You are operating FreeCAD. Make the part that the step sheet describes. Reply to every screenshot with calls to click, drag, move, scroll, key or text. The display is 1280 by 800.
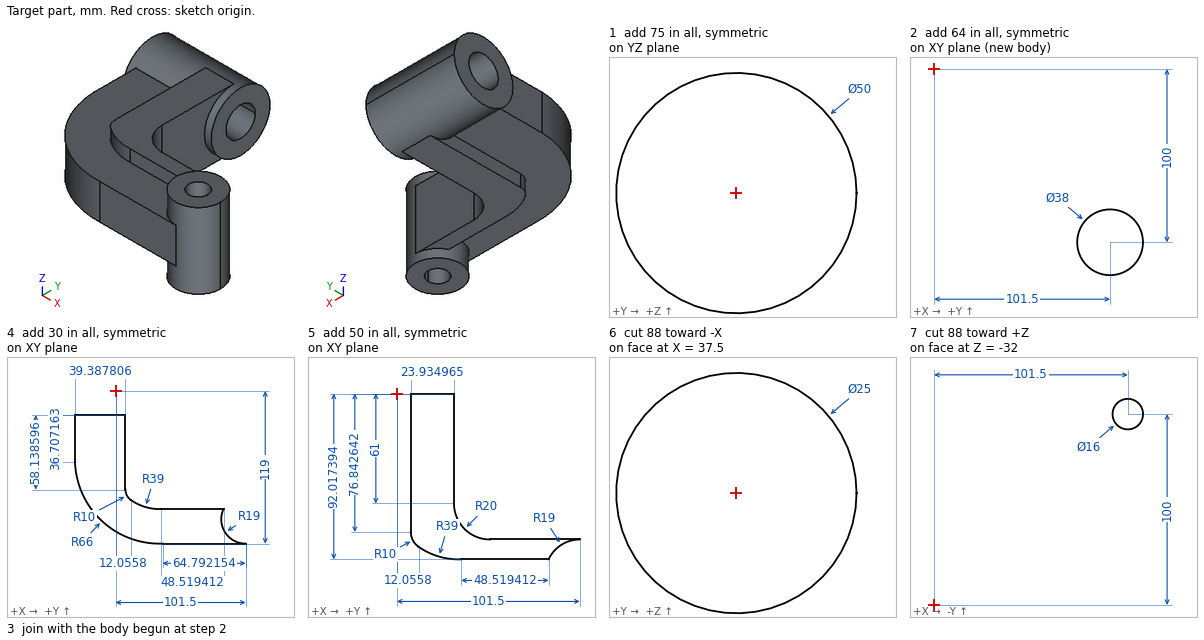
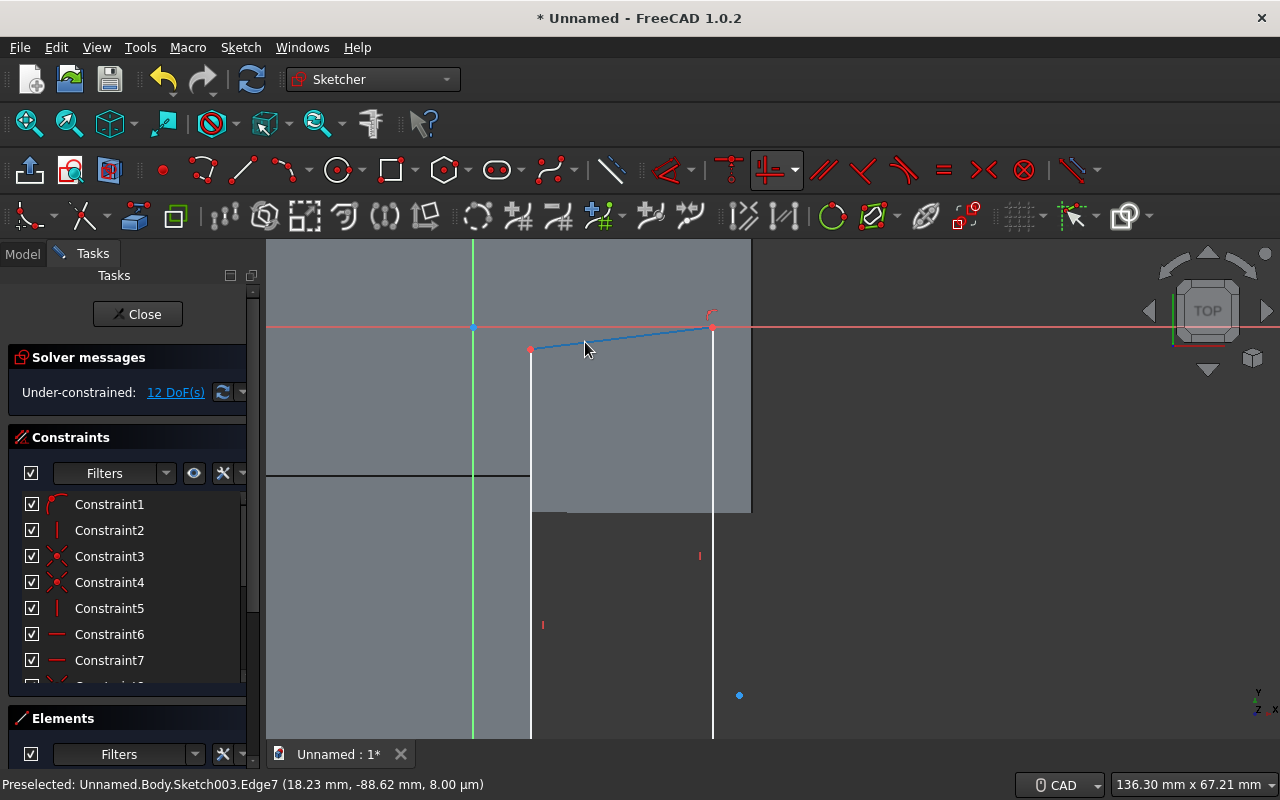
click(585, 343)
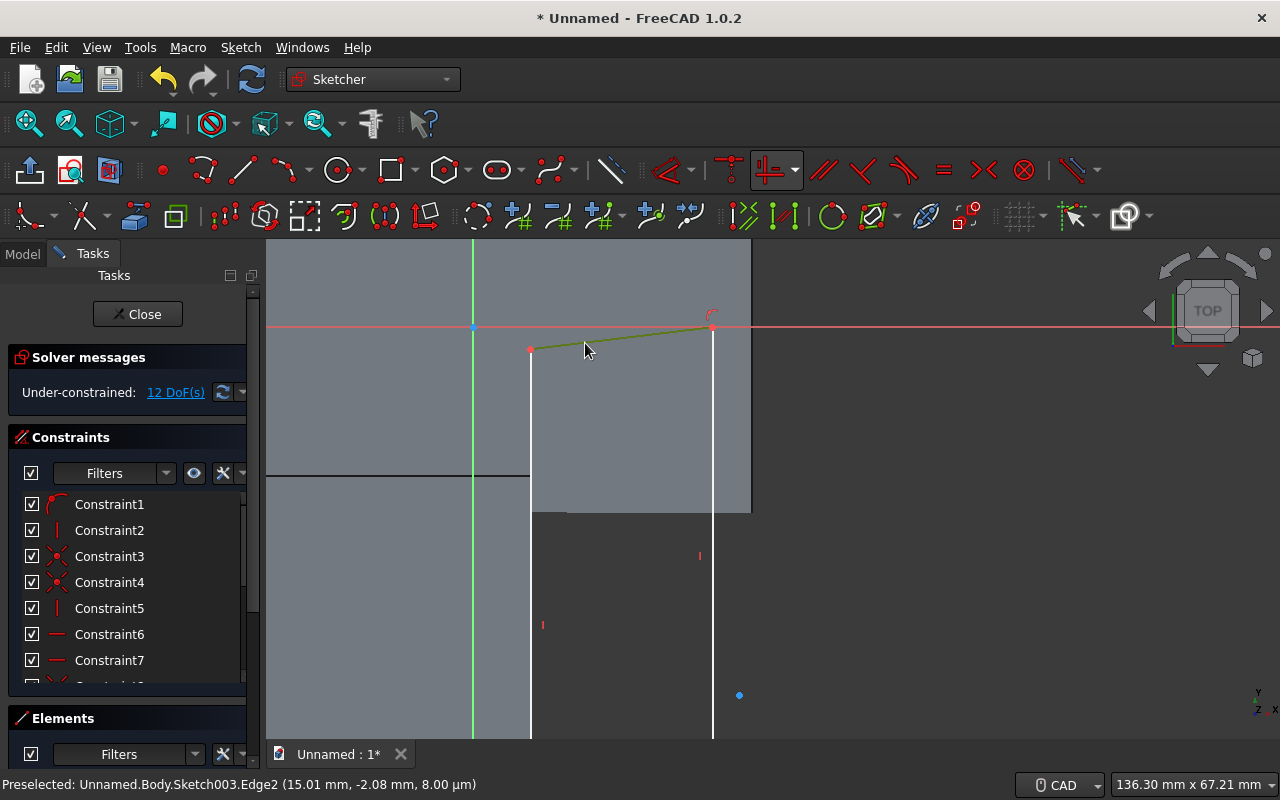
click(798, 170)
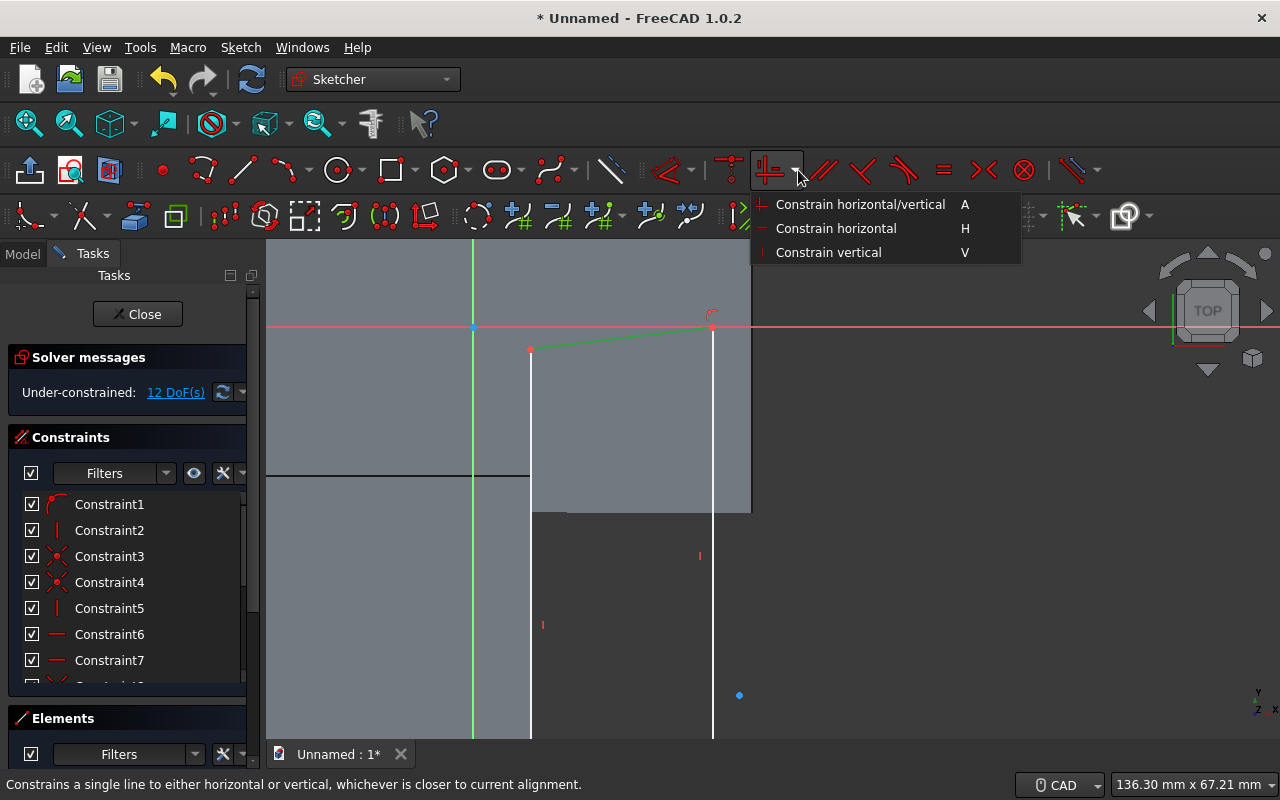
click(886, 228)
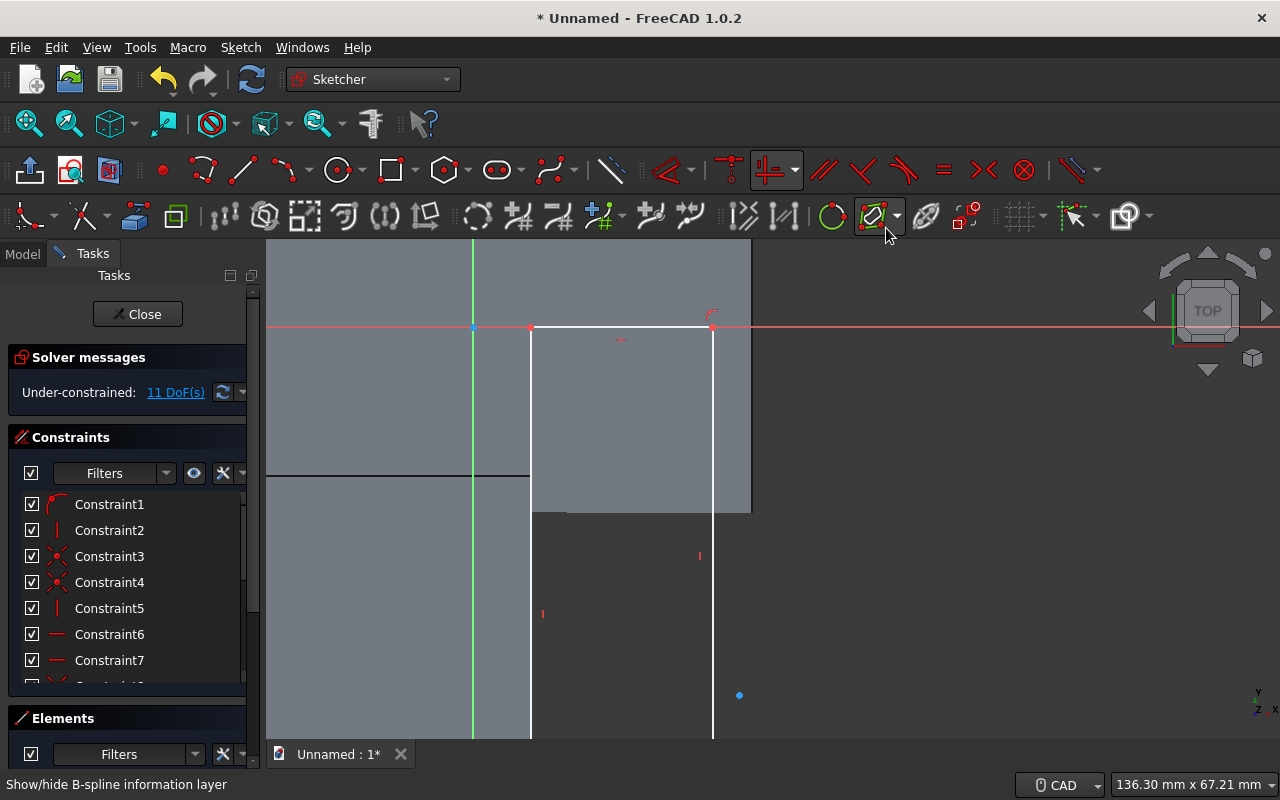
click(666, 170)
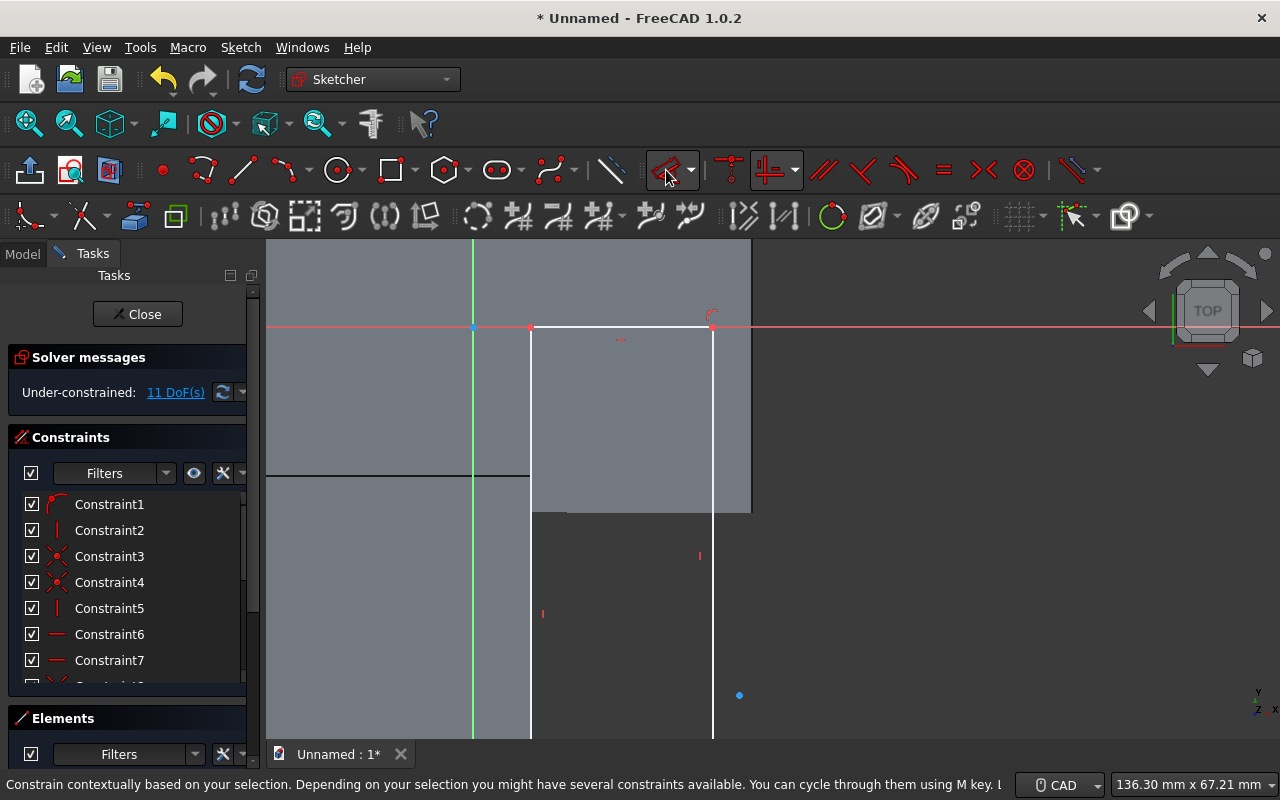
scroll(585, 342, down, 4)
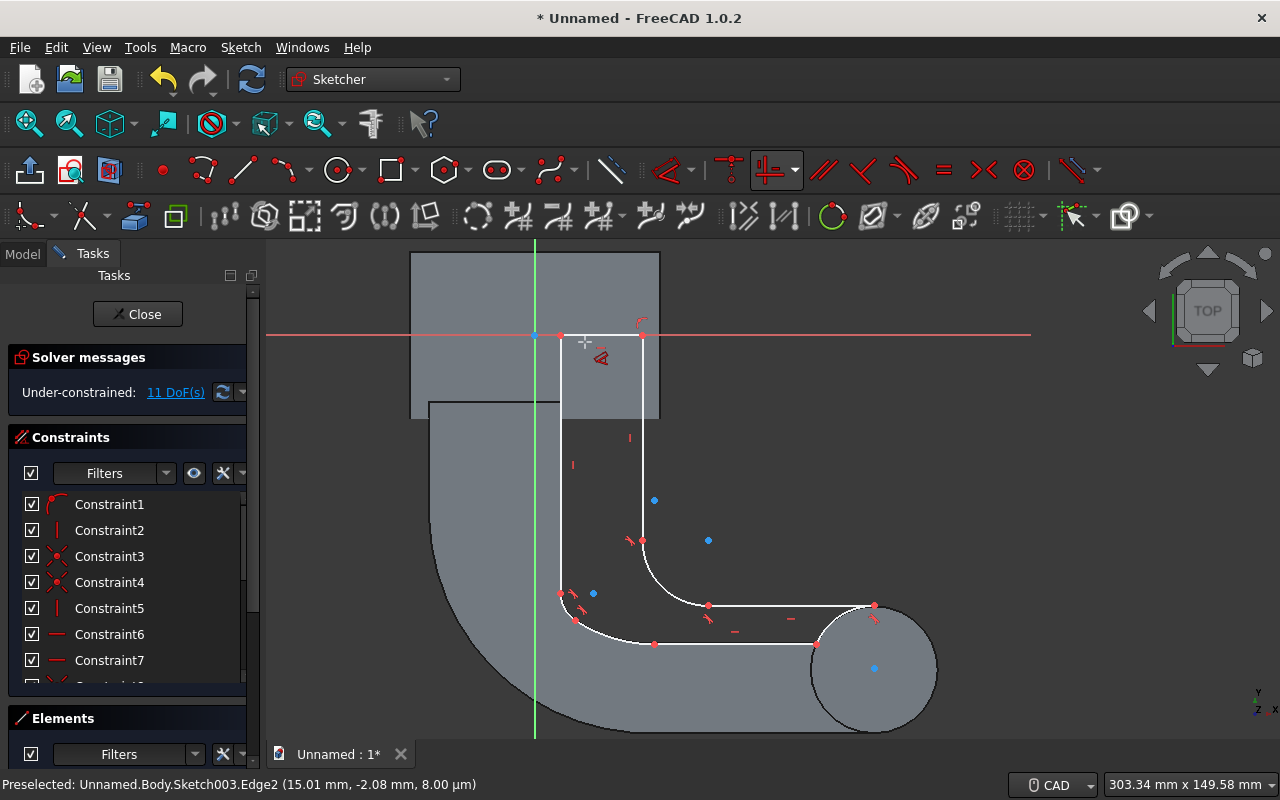
scroll(562, 603, up, 2)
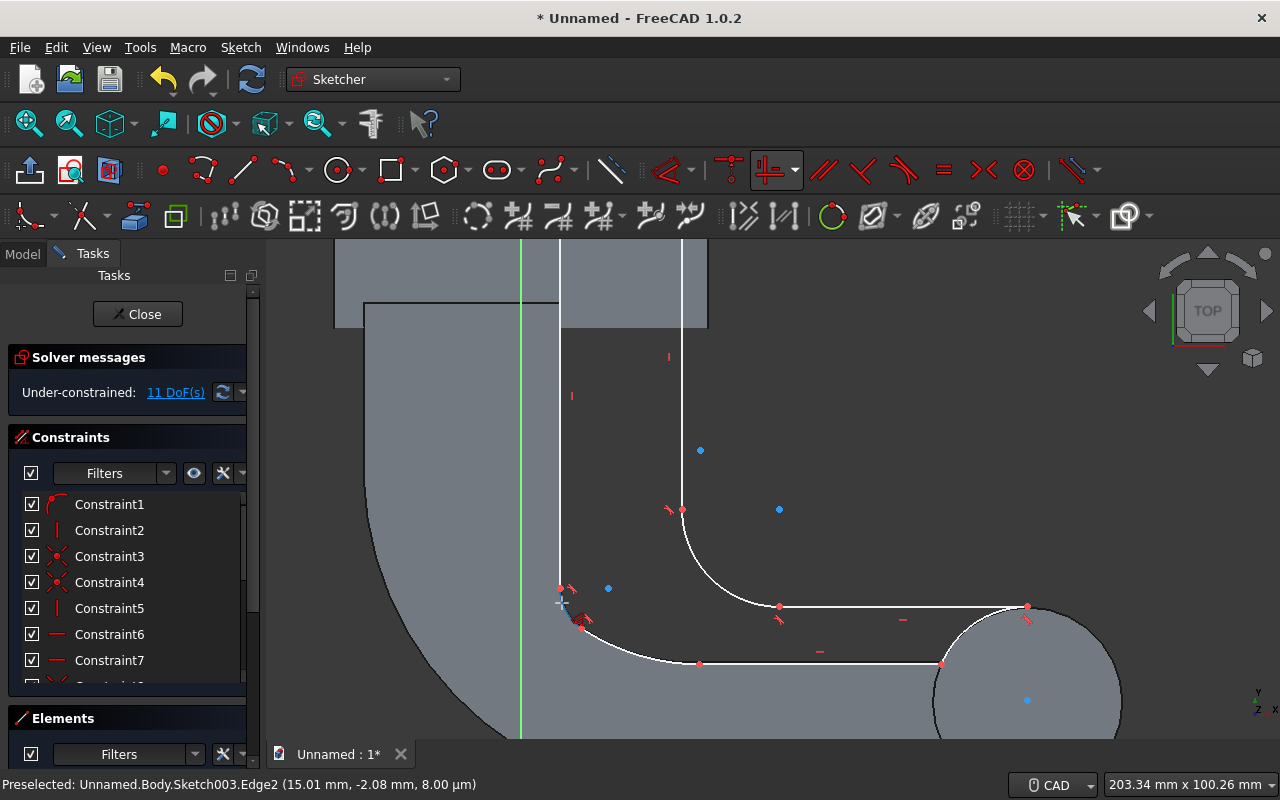
click(562, 602)
click(552, 645)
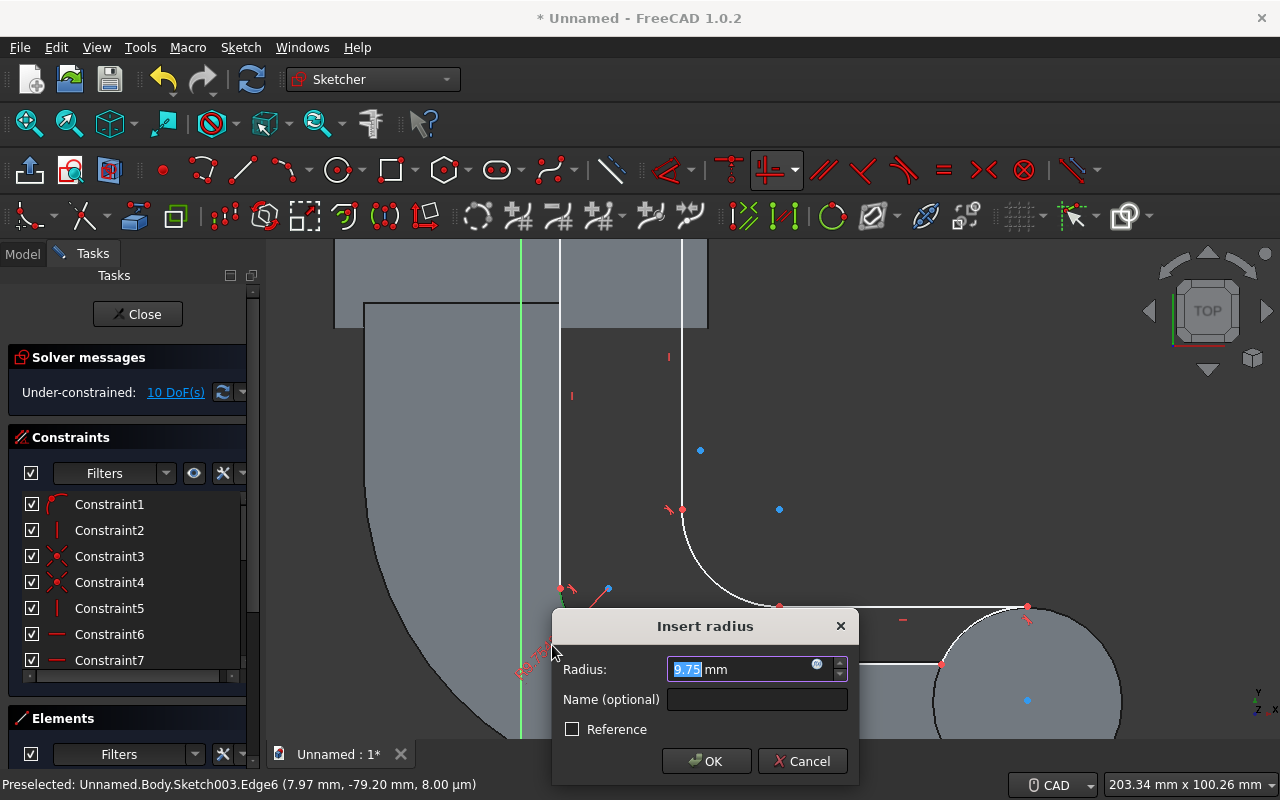
text(10)
key(Return)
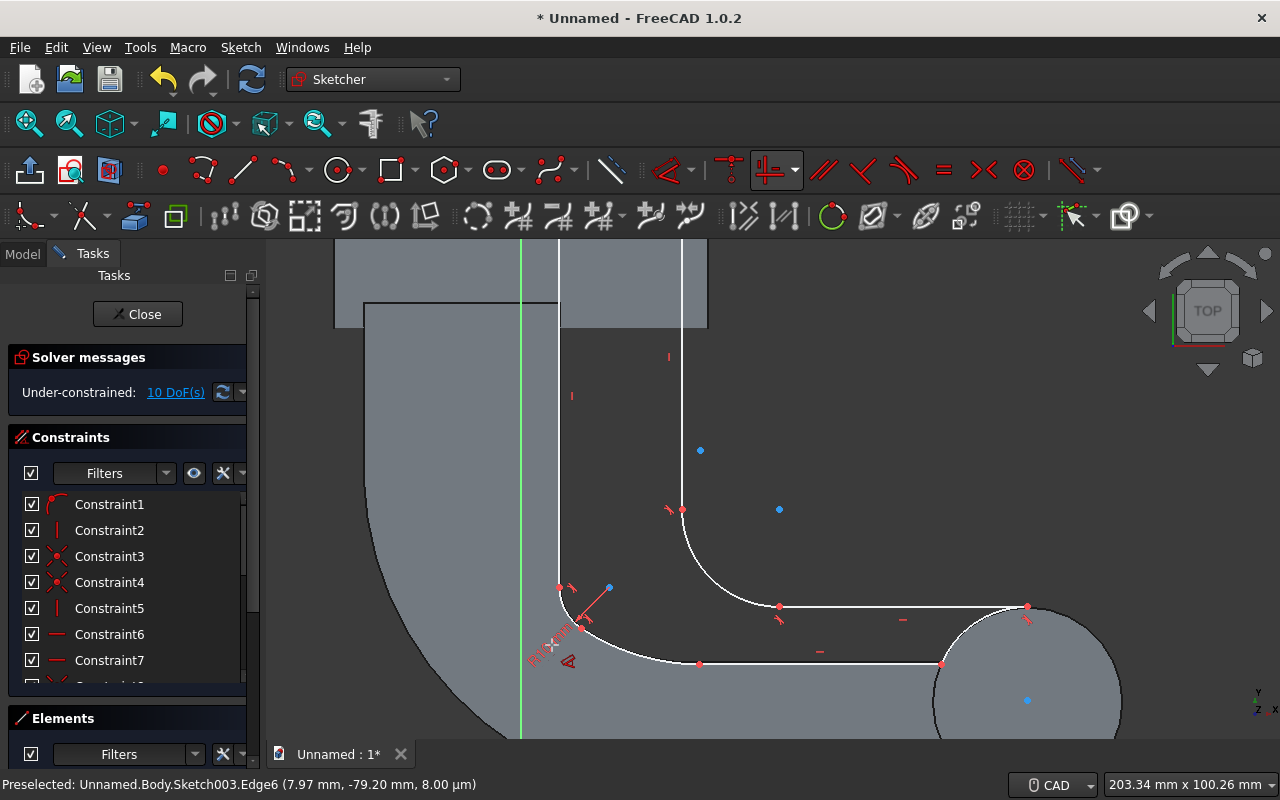
click(615, 646)
click(602, 675)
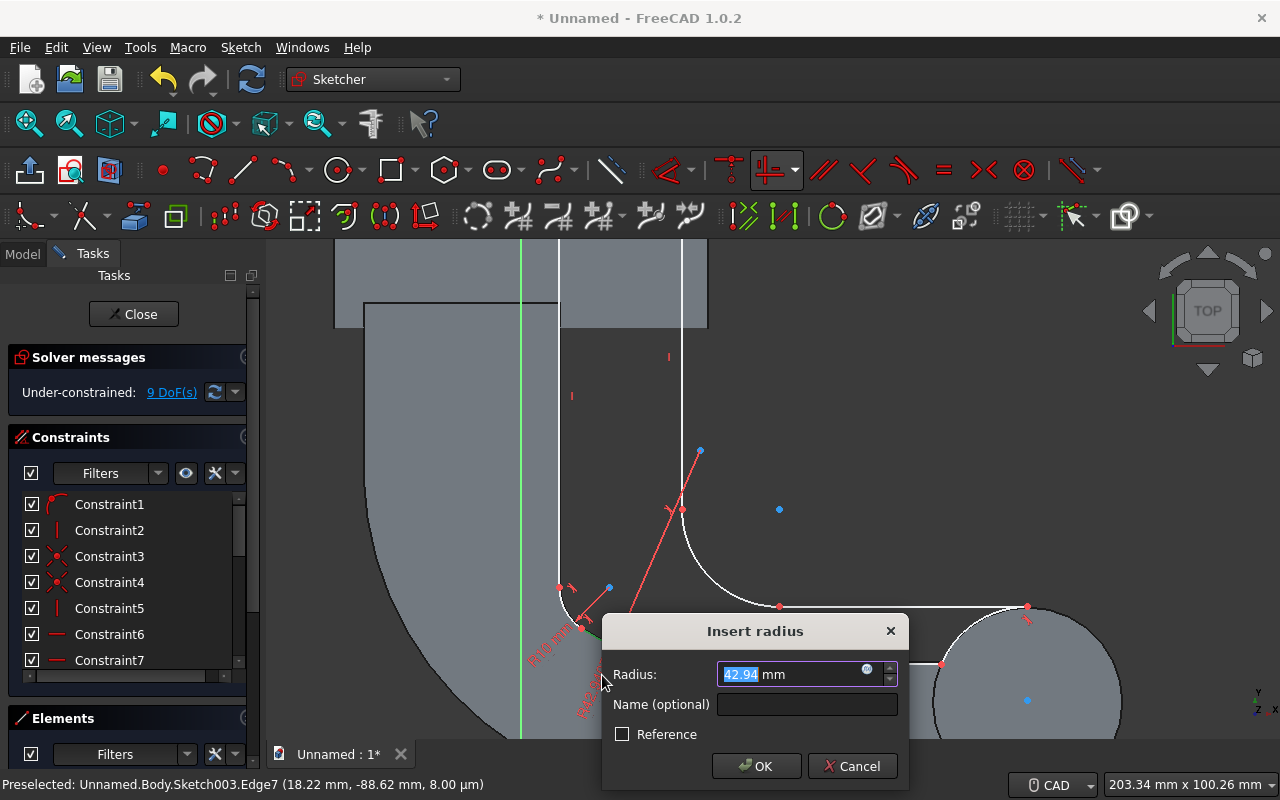
text(39)
key(Return)